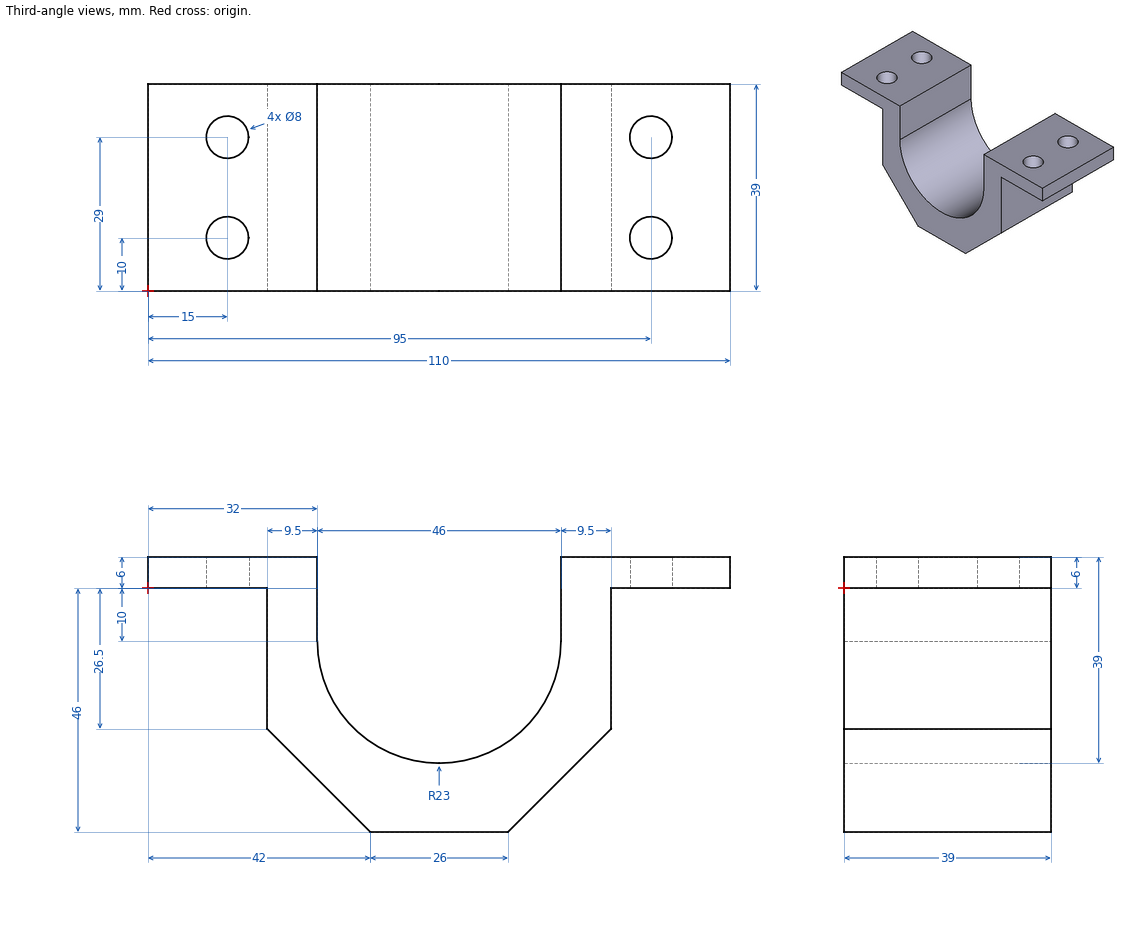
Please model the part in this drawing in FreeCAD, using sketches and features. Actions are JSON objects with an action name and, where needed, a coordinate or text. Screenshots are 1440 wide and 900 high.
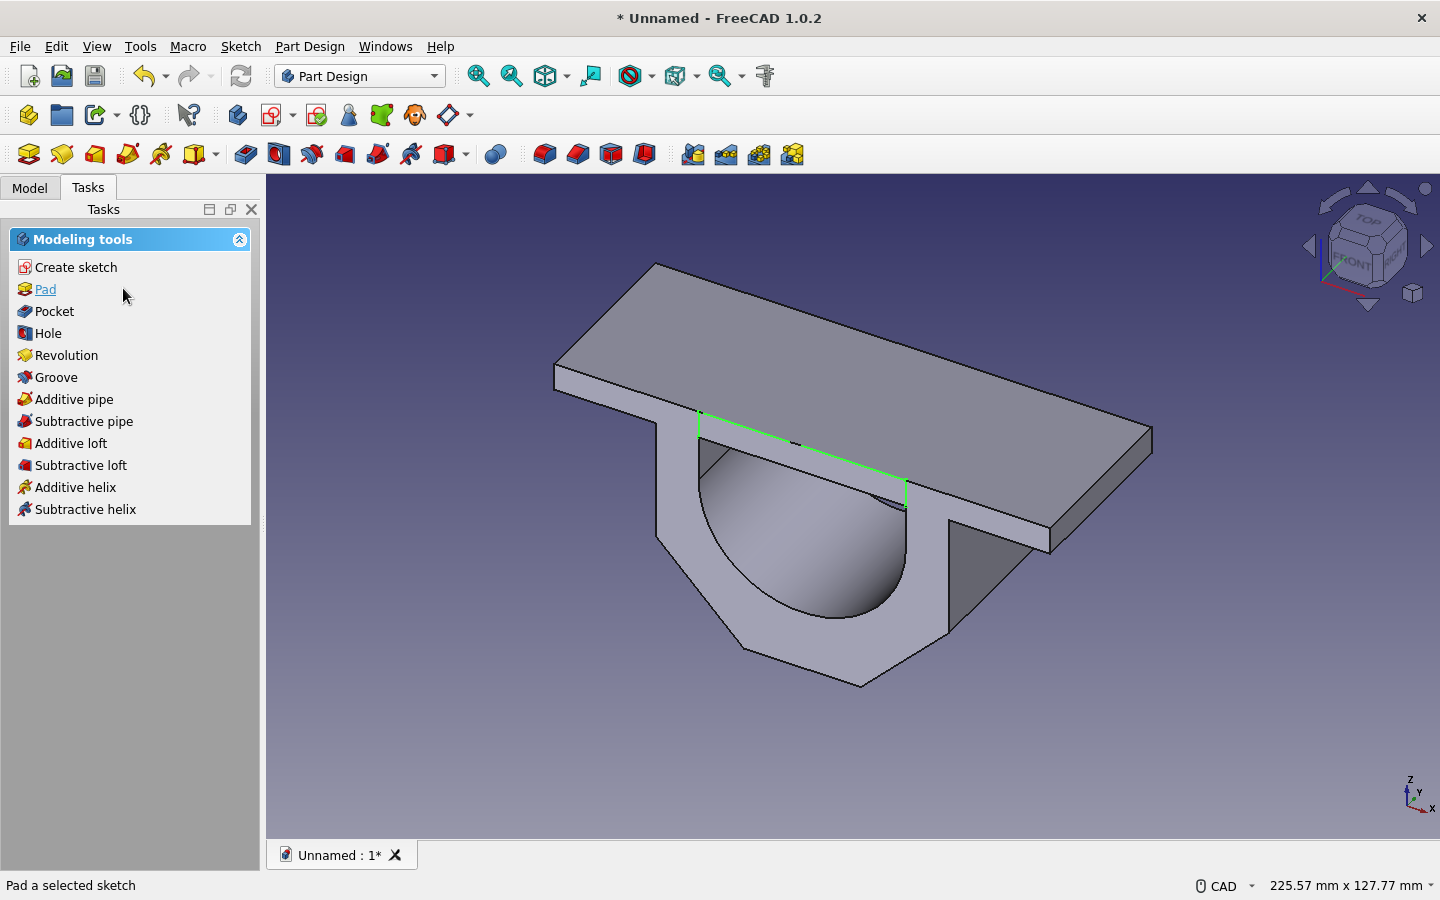
{"action": "left_click", "coordinate": [246, 154]}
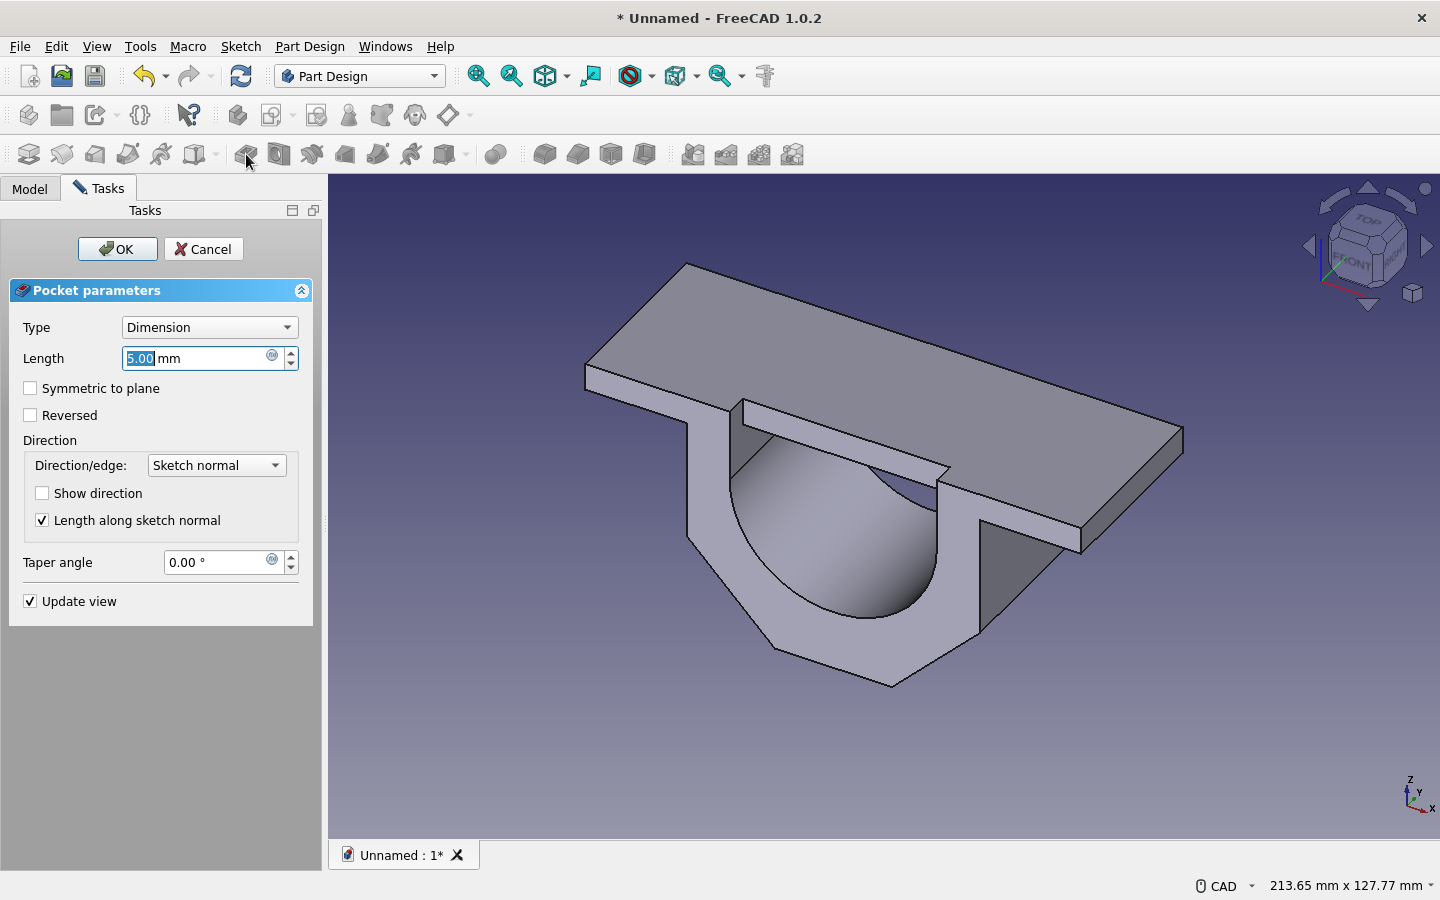
{"action": "type", "text": "39"}
{"action": "key", "text": "Tab"}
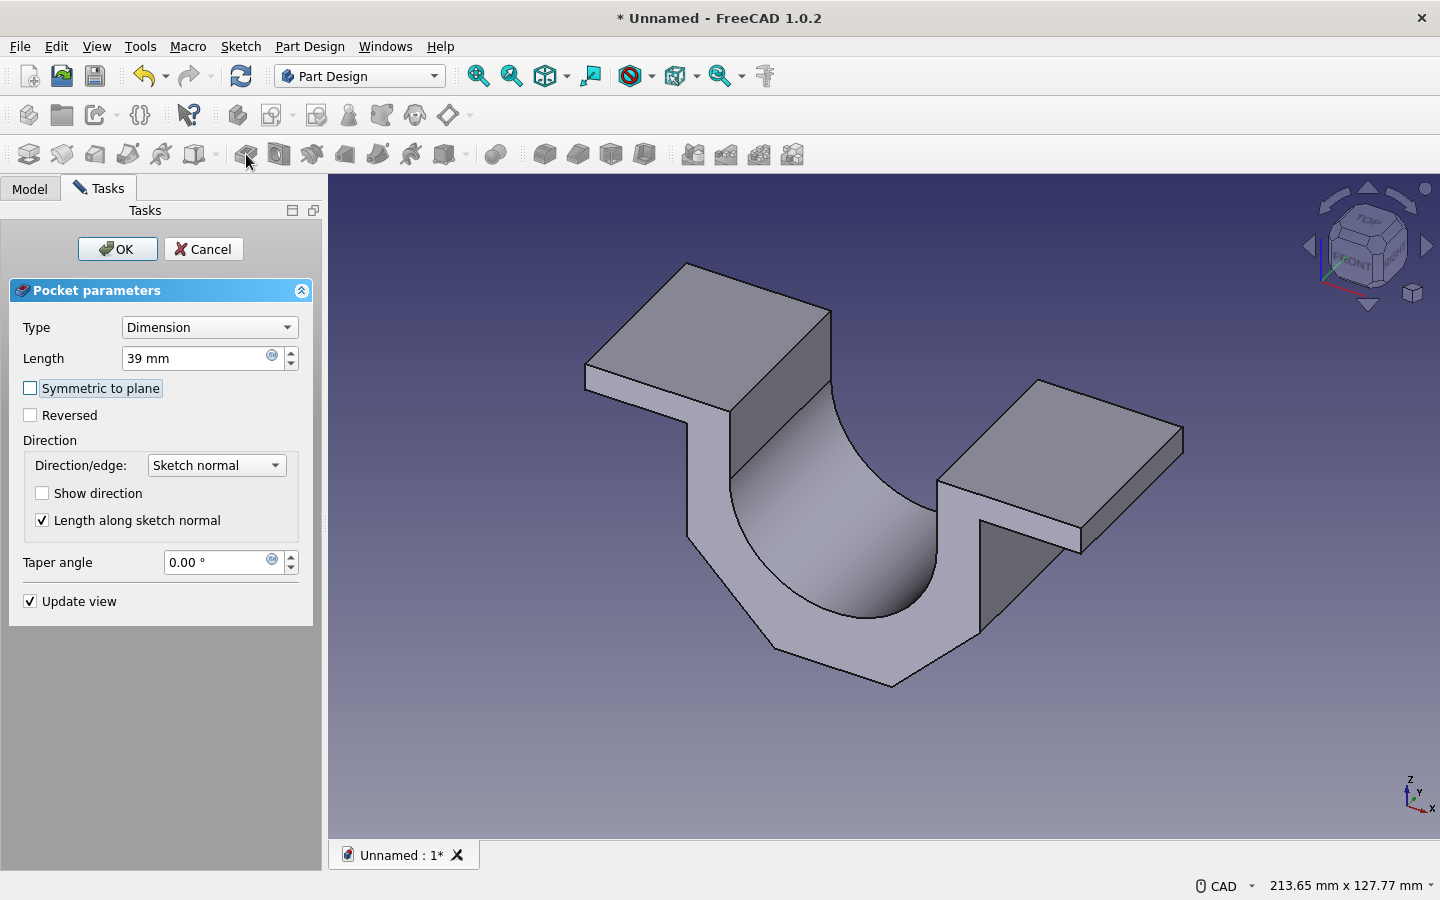
{"action": "left_click", "coordinate": [118, 249]}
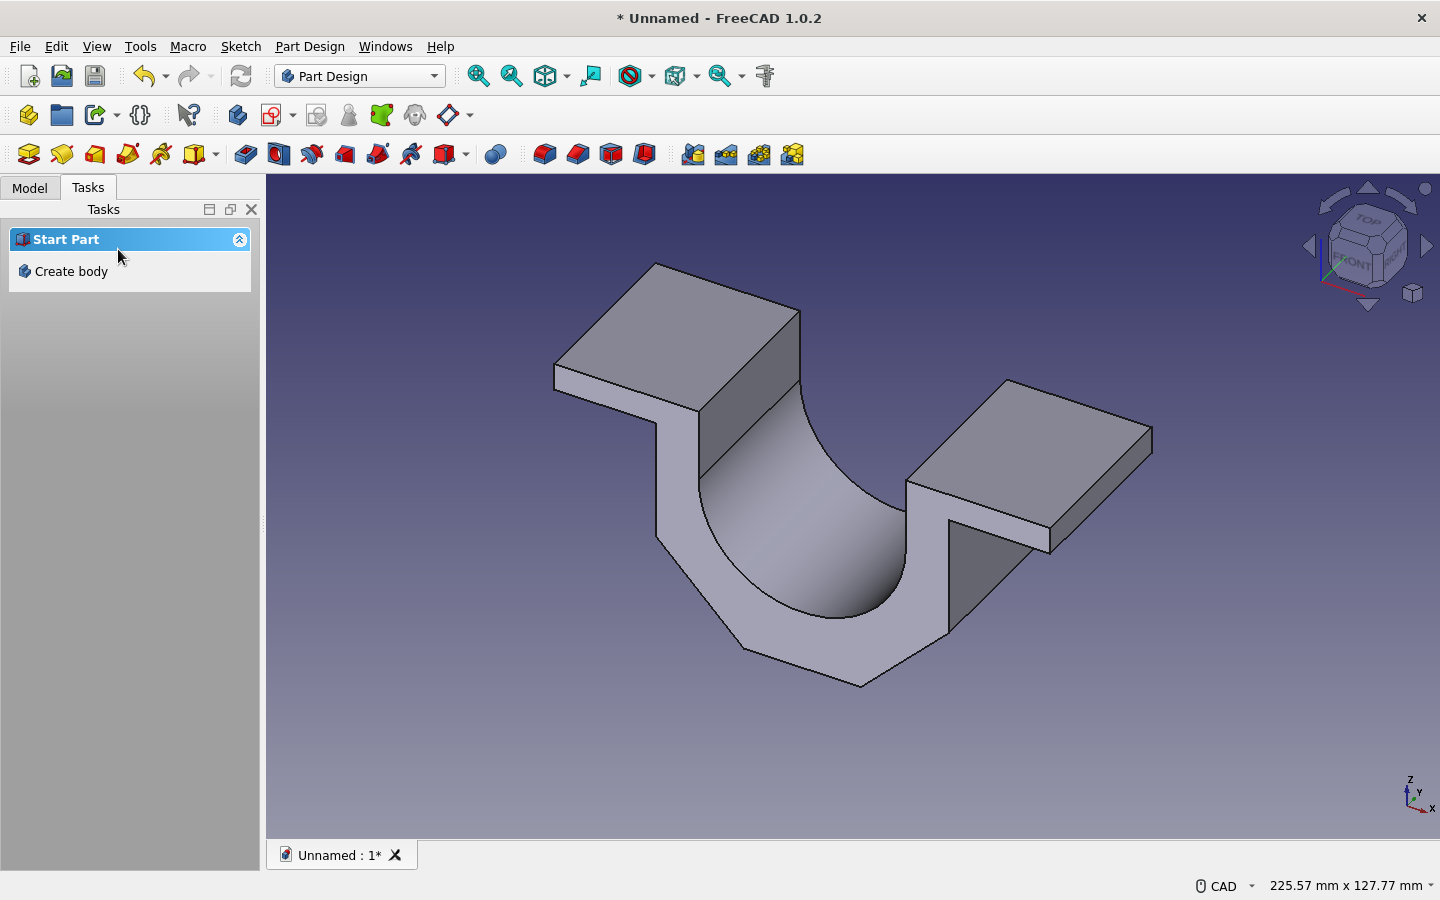
{"action": "left_click", "coordinate": [677, 336]}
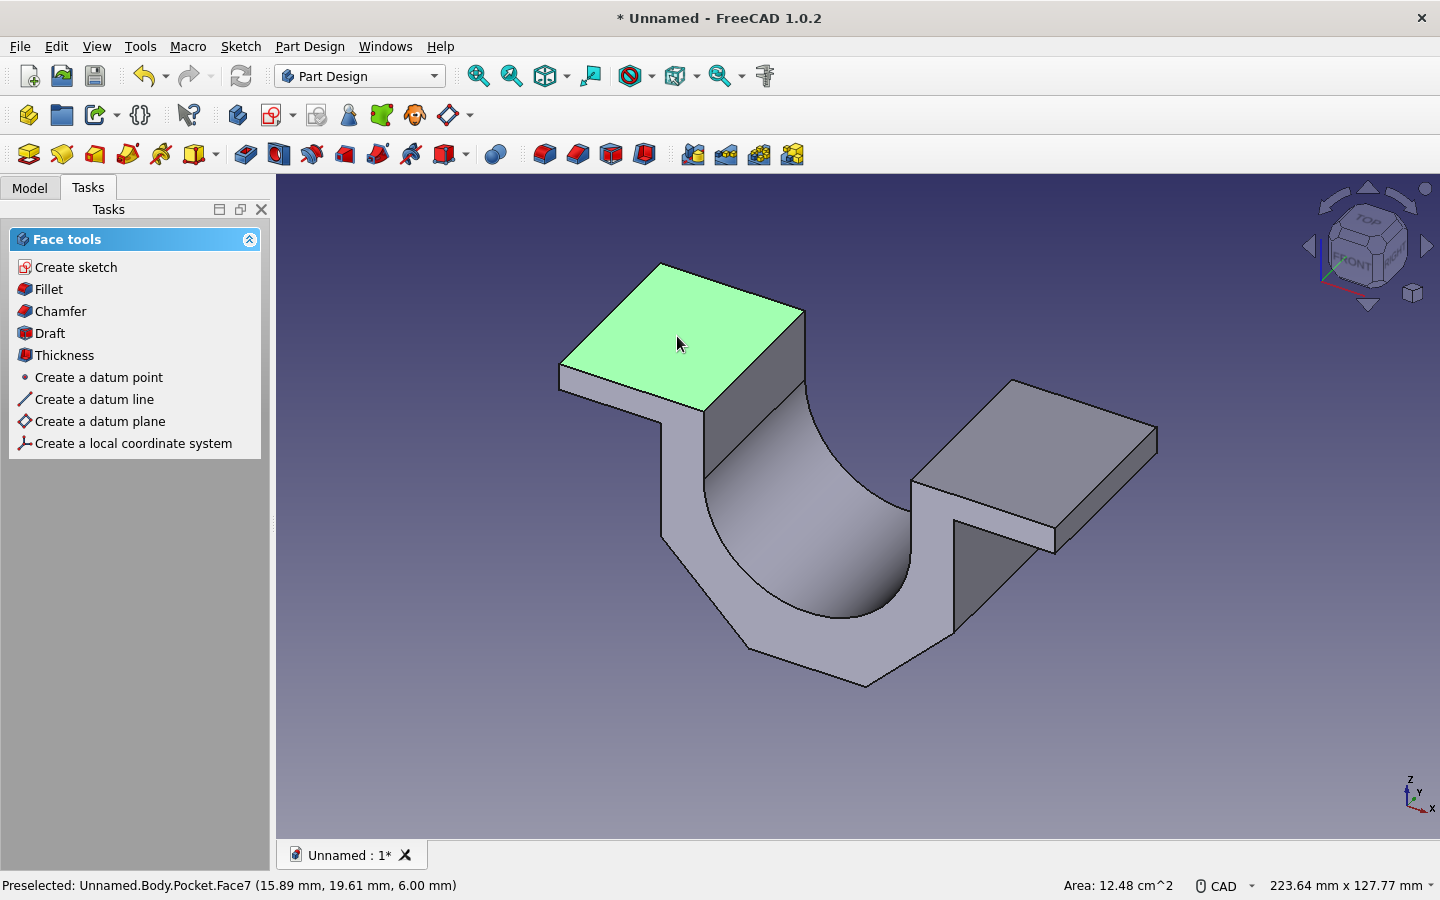
{"action": "left_click", "coordinate": [270, 116]}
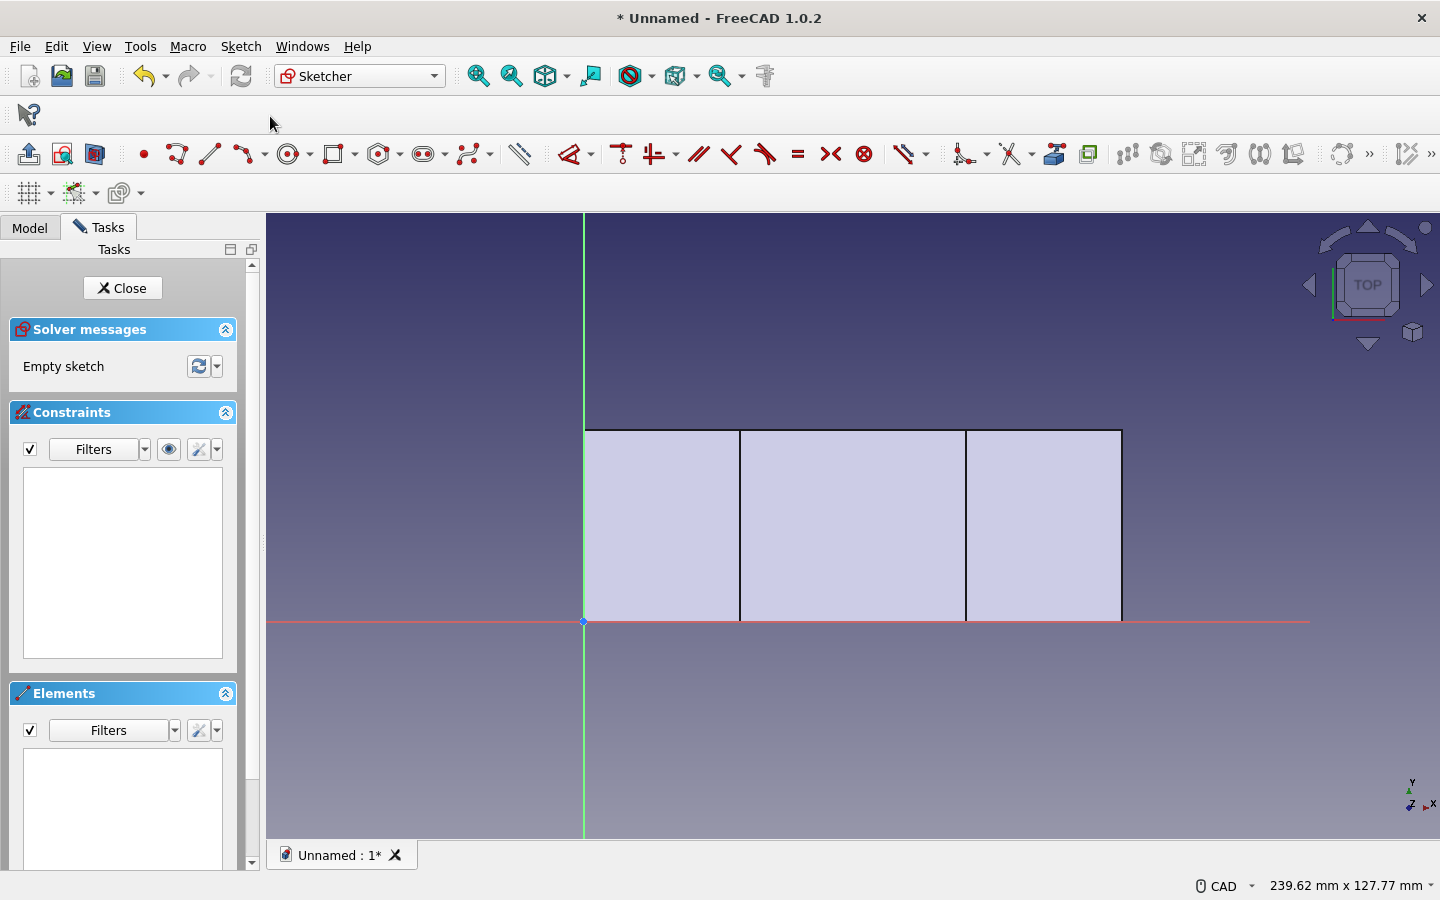
{"action": "scroll", "coordinate": [911, 571], "scroll_direction": "up", "scroll_amount": 2}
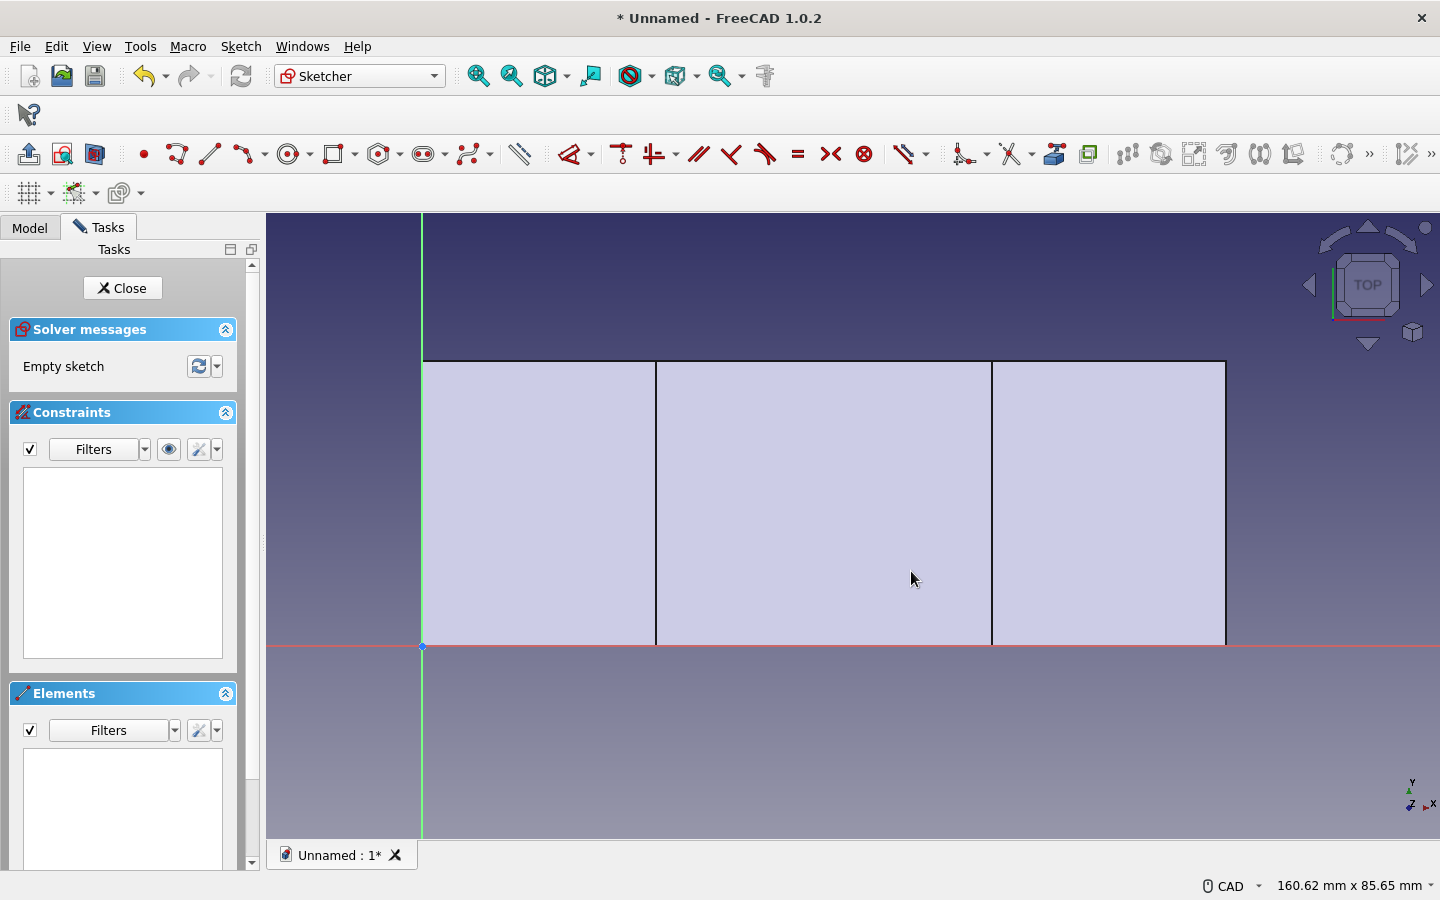
{"action": "key", "text": "g c"}